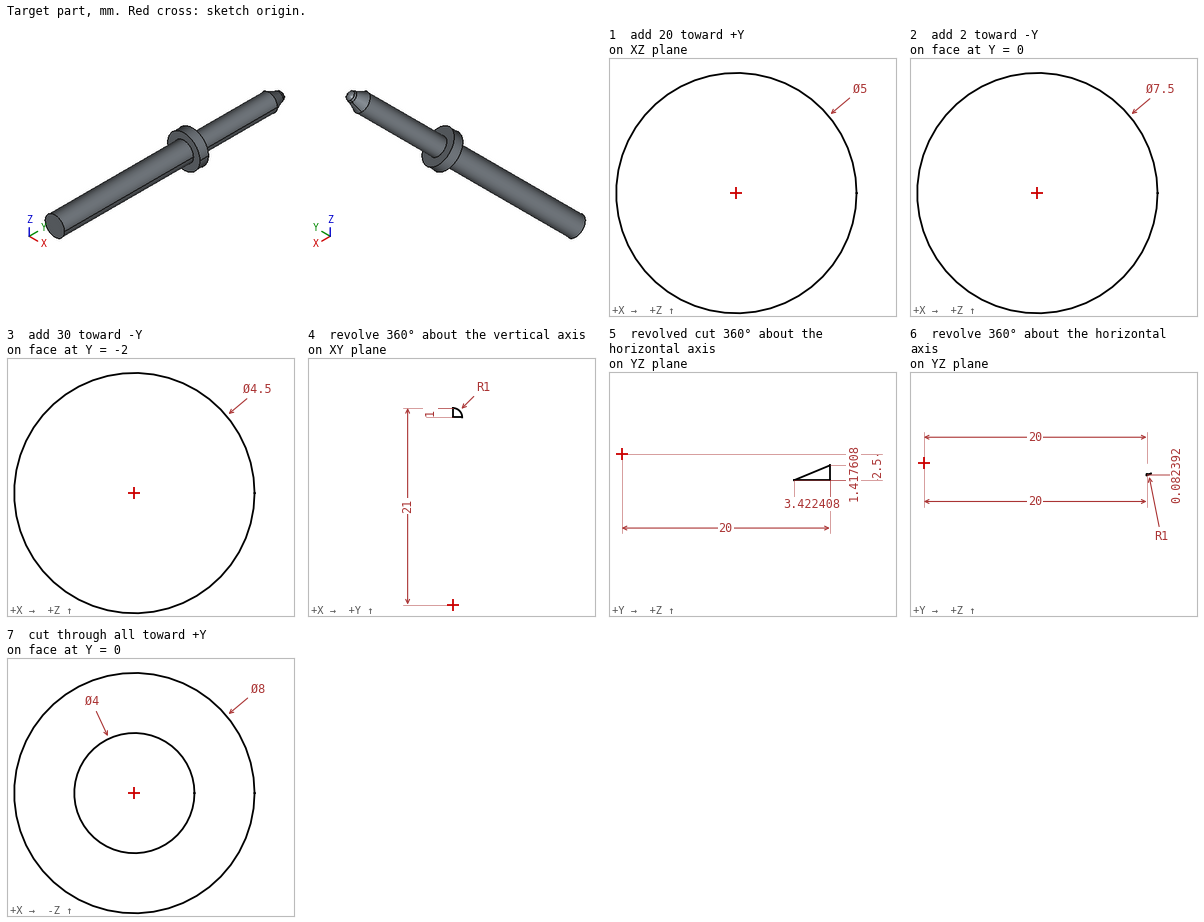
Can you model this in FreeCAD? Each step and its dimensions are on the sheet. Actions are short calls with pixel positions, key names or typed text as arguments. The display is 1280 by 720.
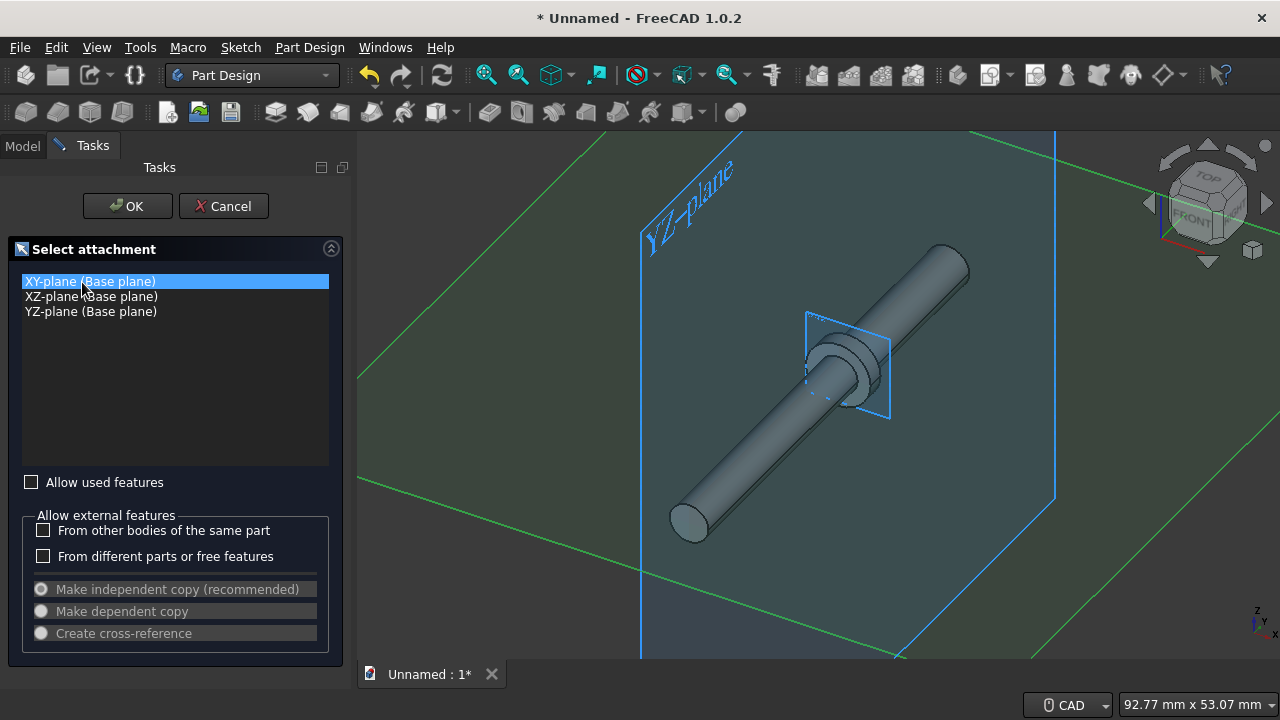
click(128, 206)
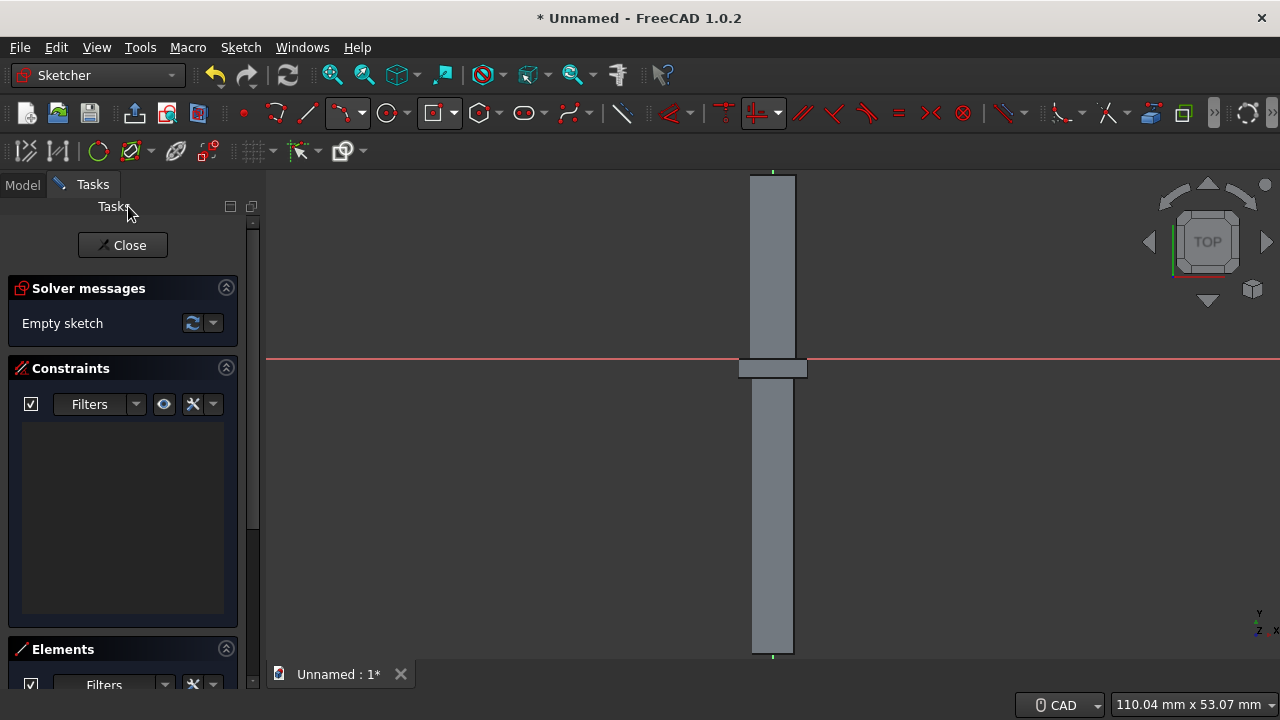
click(200, 114)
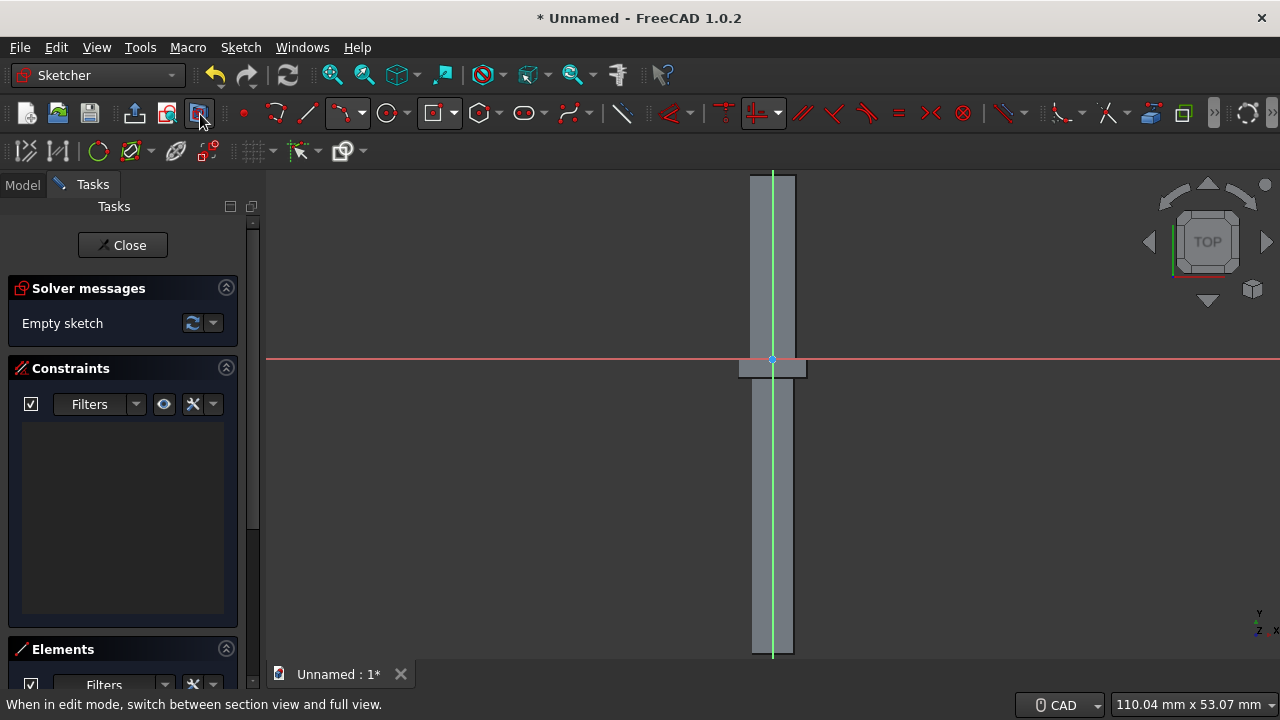
scroll(704, 414, down, 5)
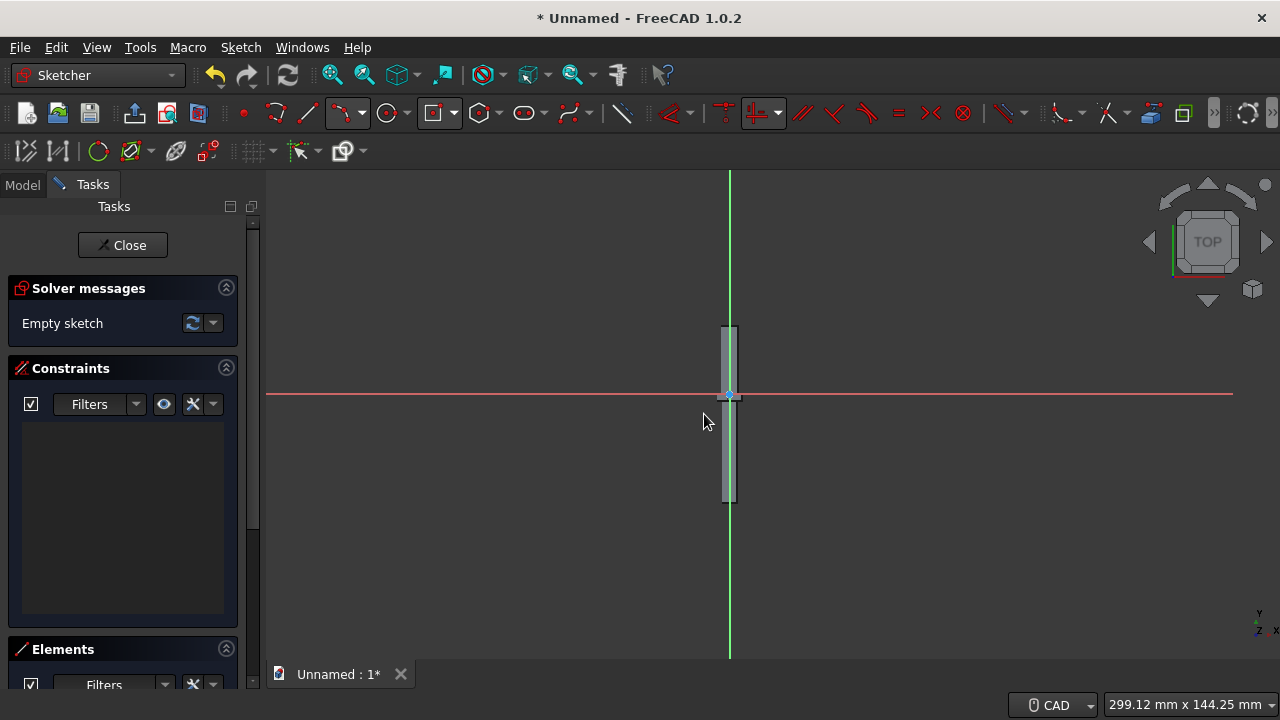
scroll(733, 320, up, 15)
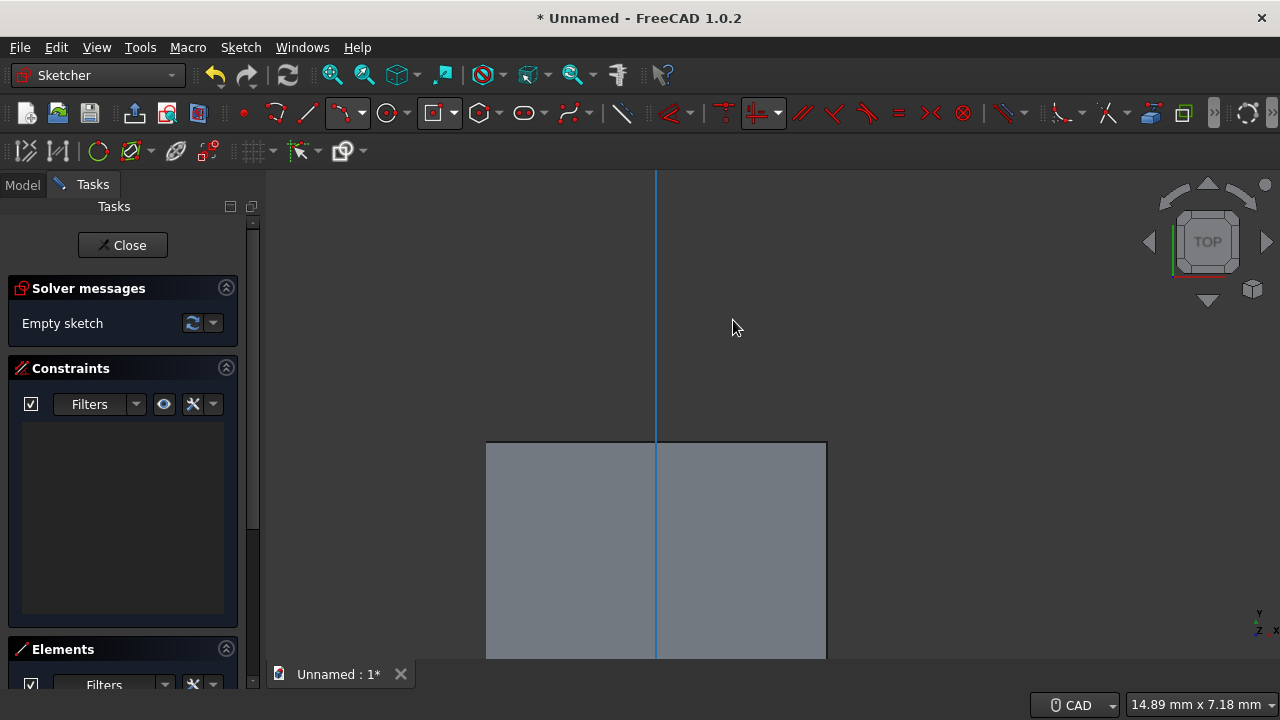
scroll(687, 406, up, 8)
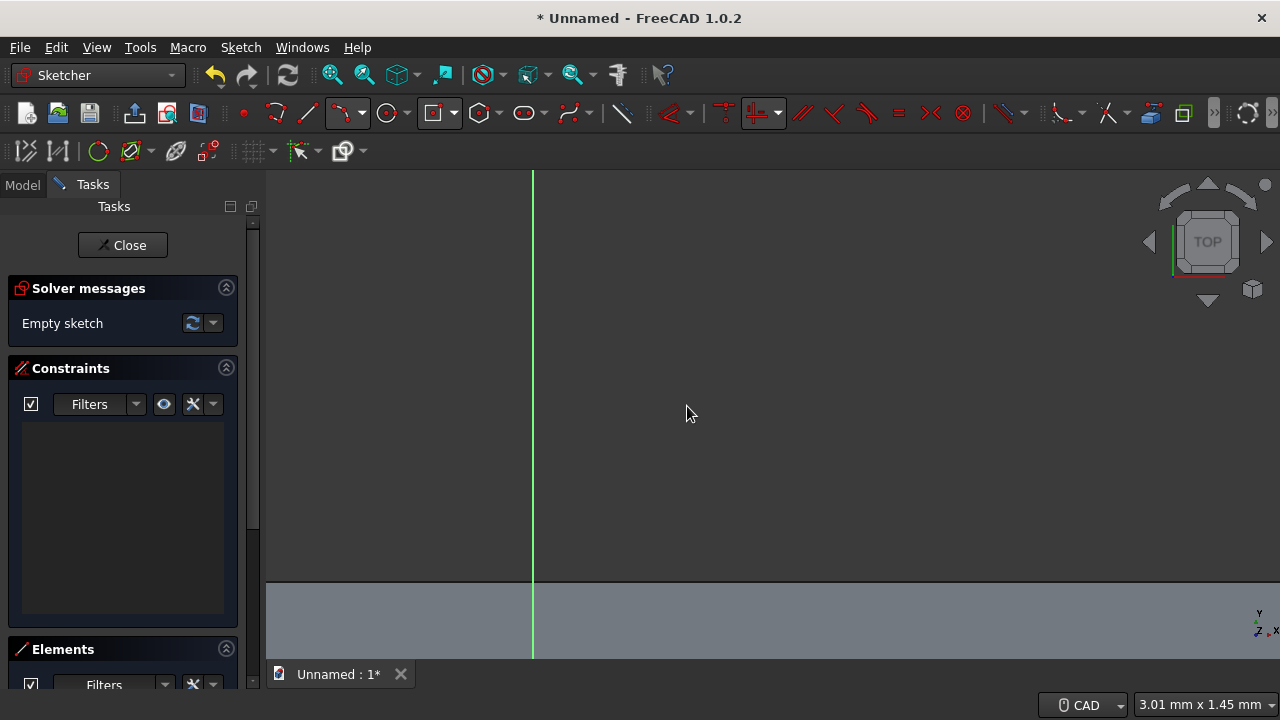
click(276, 114)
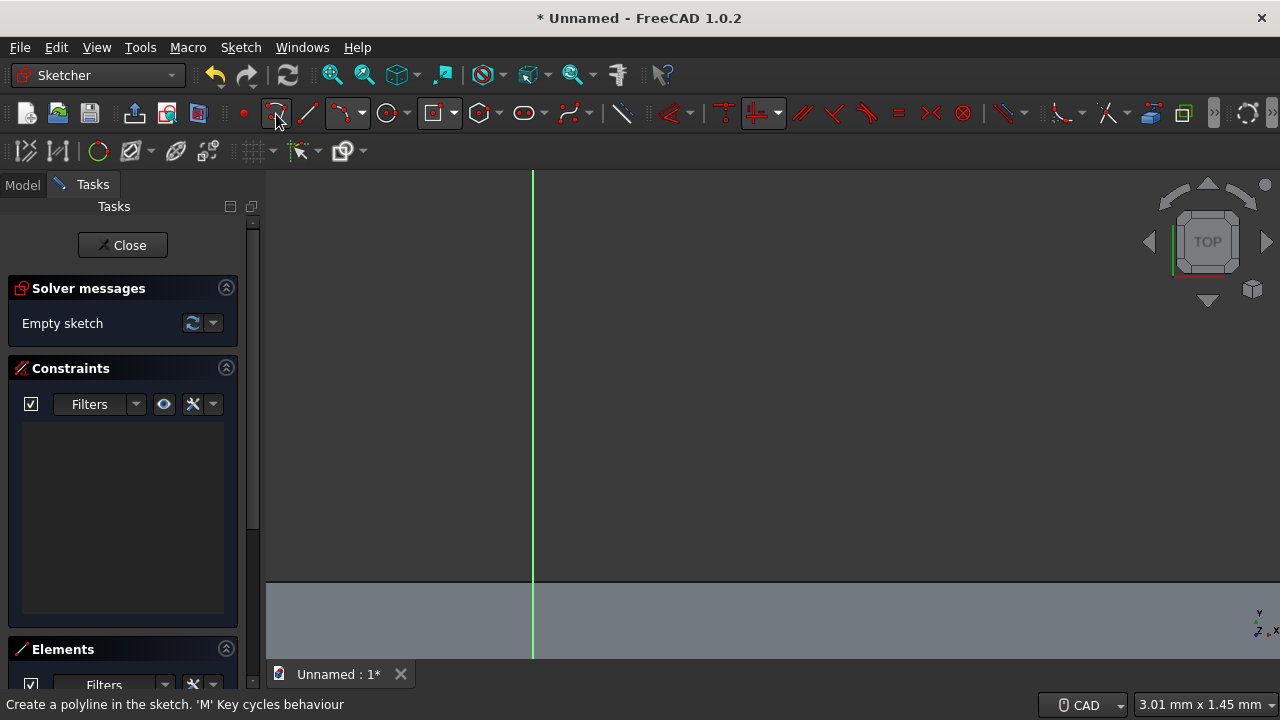
click(533, 245)
click(542, 582)
click(871, 582)
right_click(871, 582)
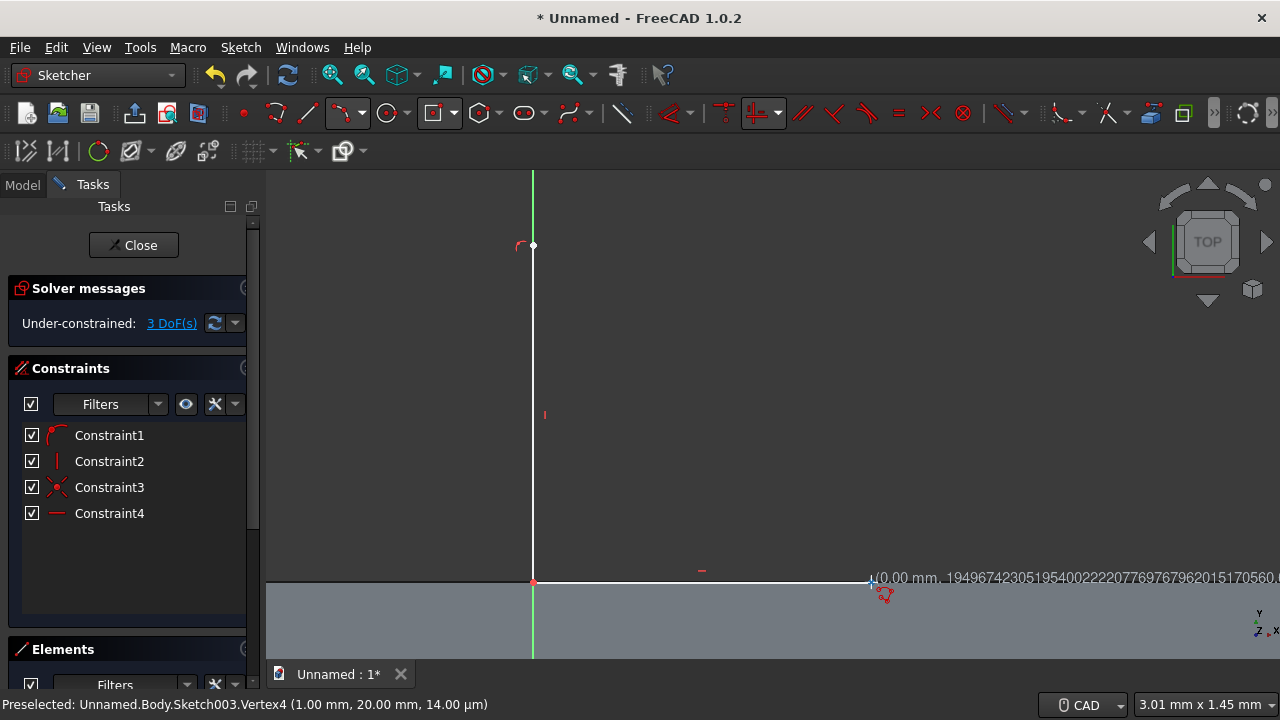
click(342, 114)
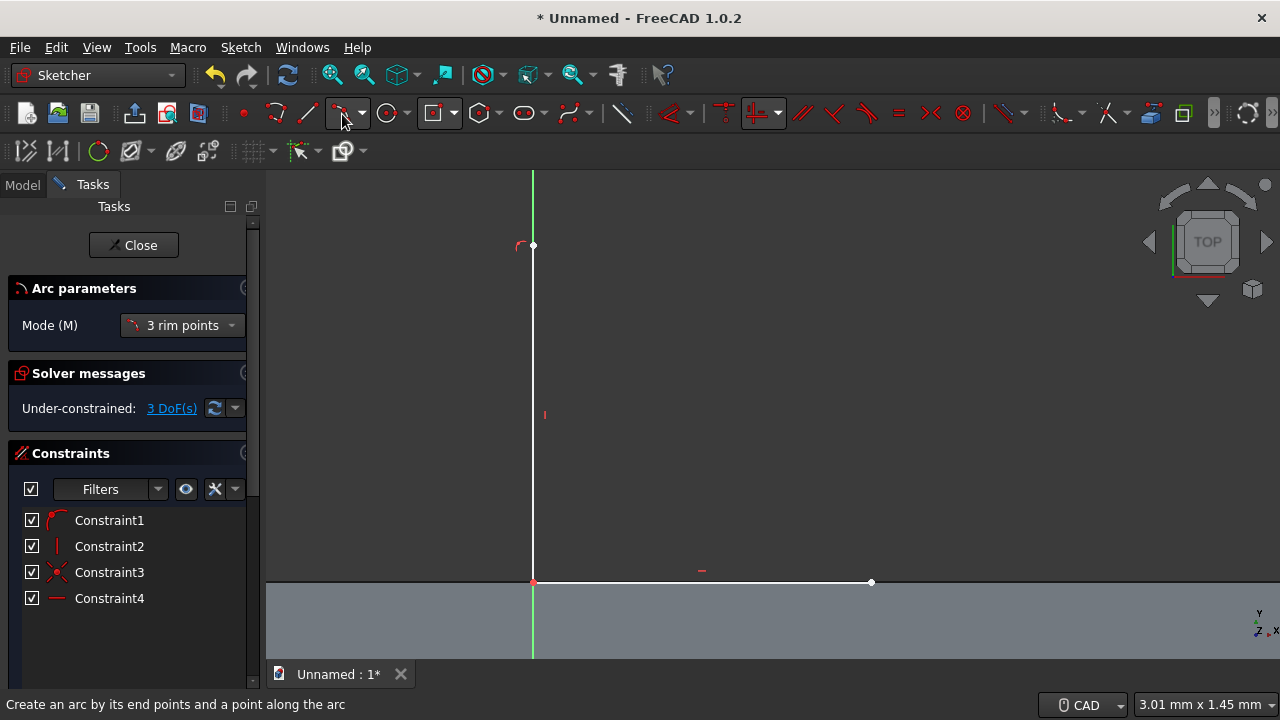
click(871, 583)
click(533, 246)
click(772, 343)
key(Escape)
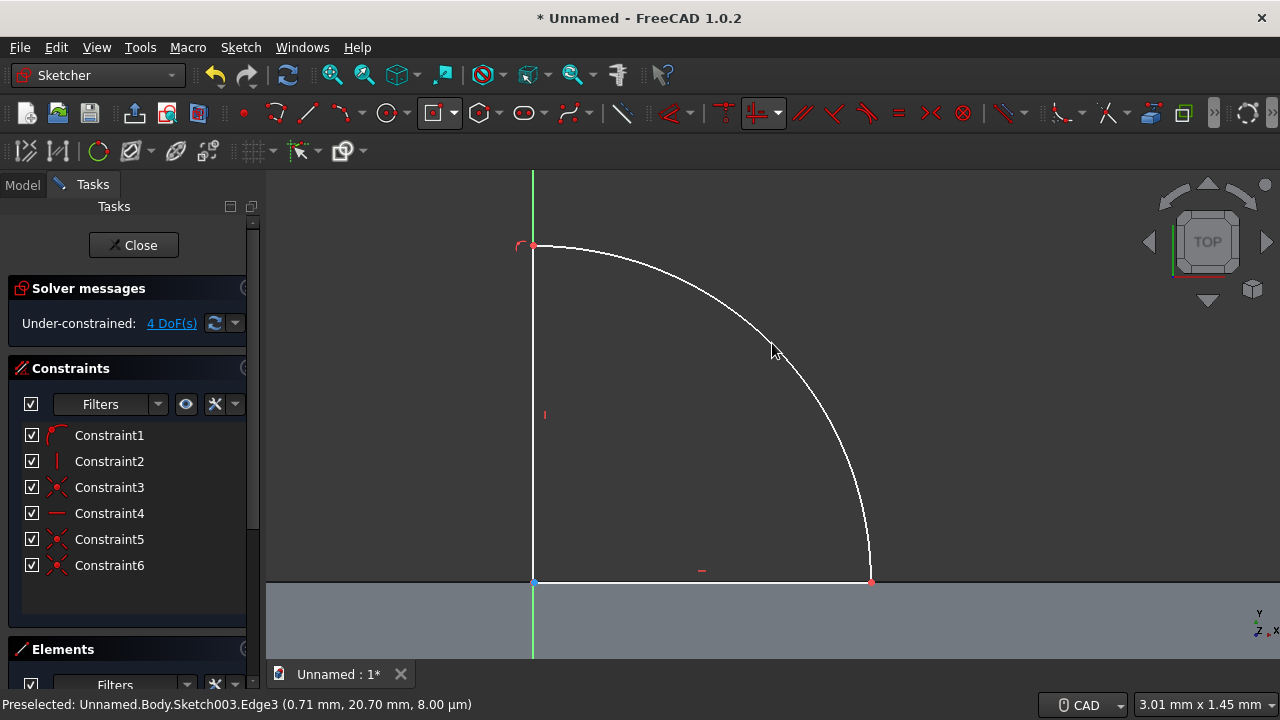
click(535, 582)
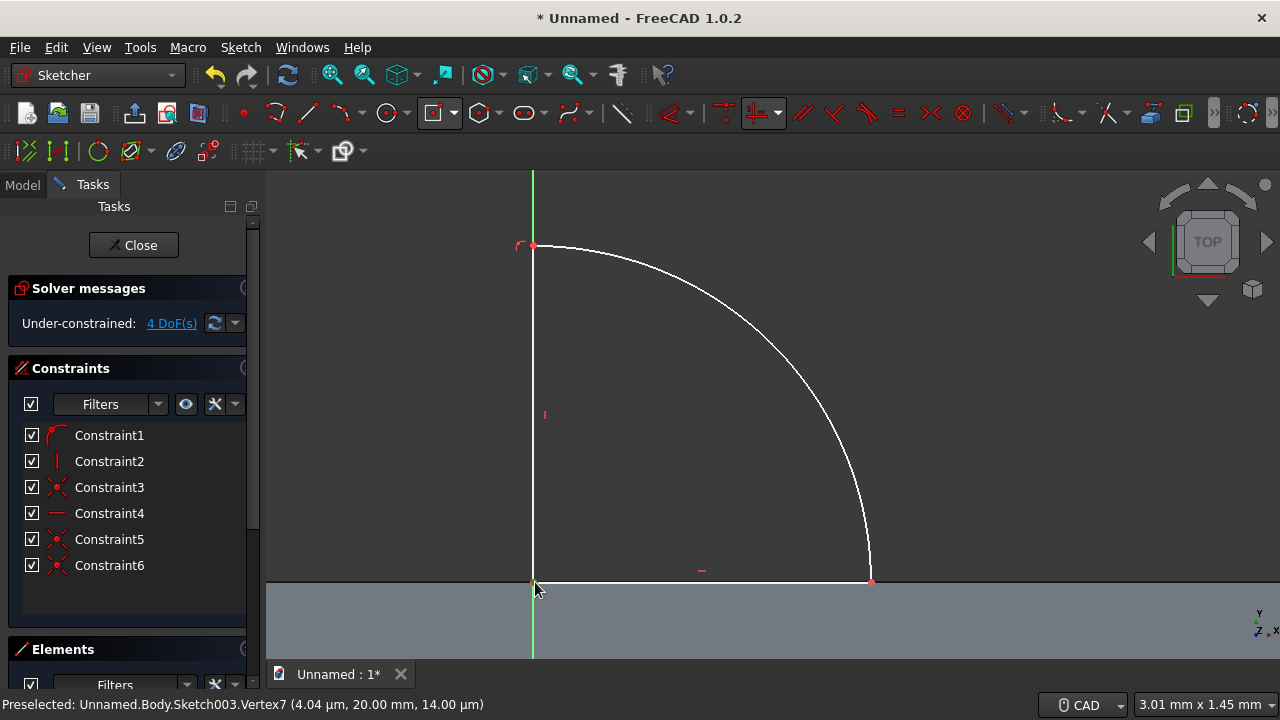
click(533, 600)